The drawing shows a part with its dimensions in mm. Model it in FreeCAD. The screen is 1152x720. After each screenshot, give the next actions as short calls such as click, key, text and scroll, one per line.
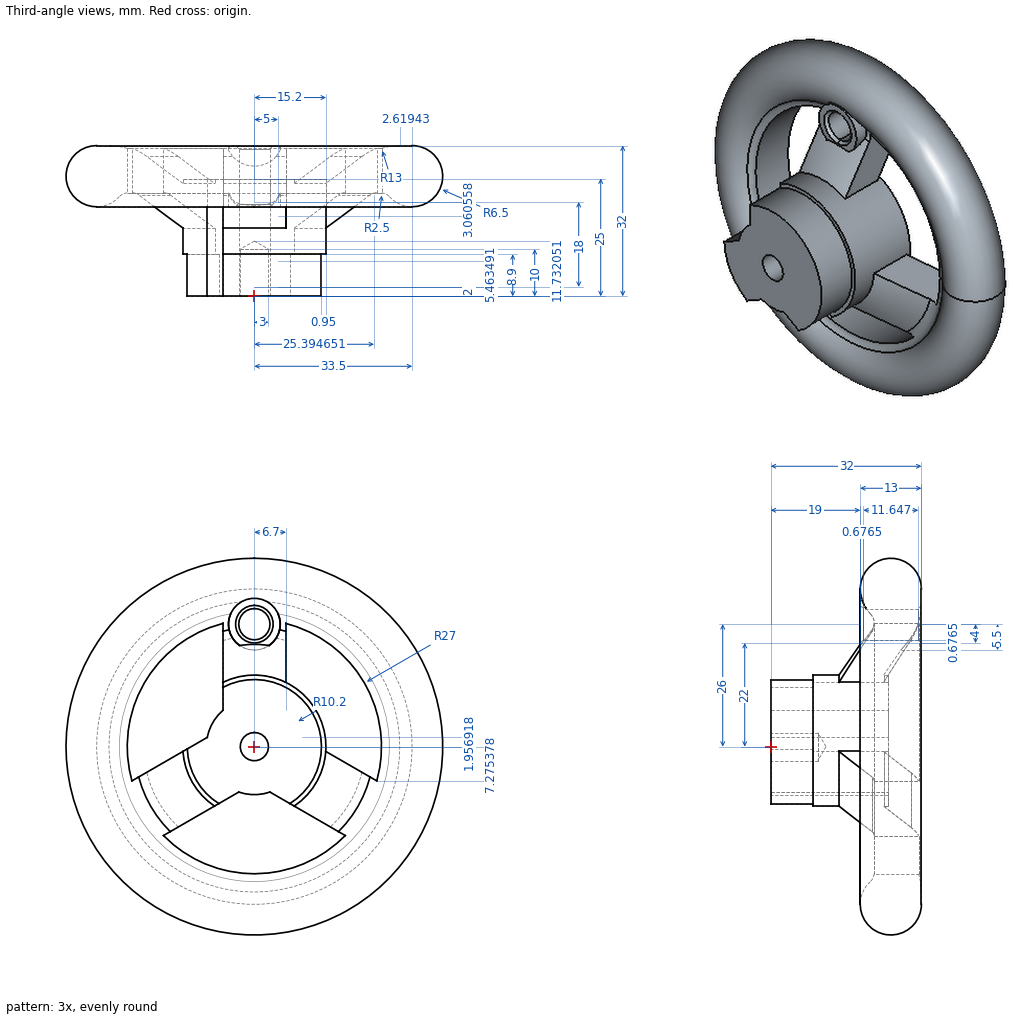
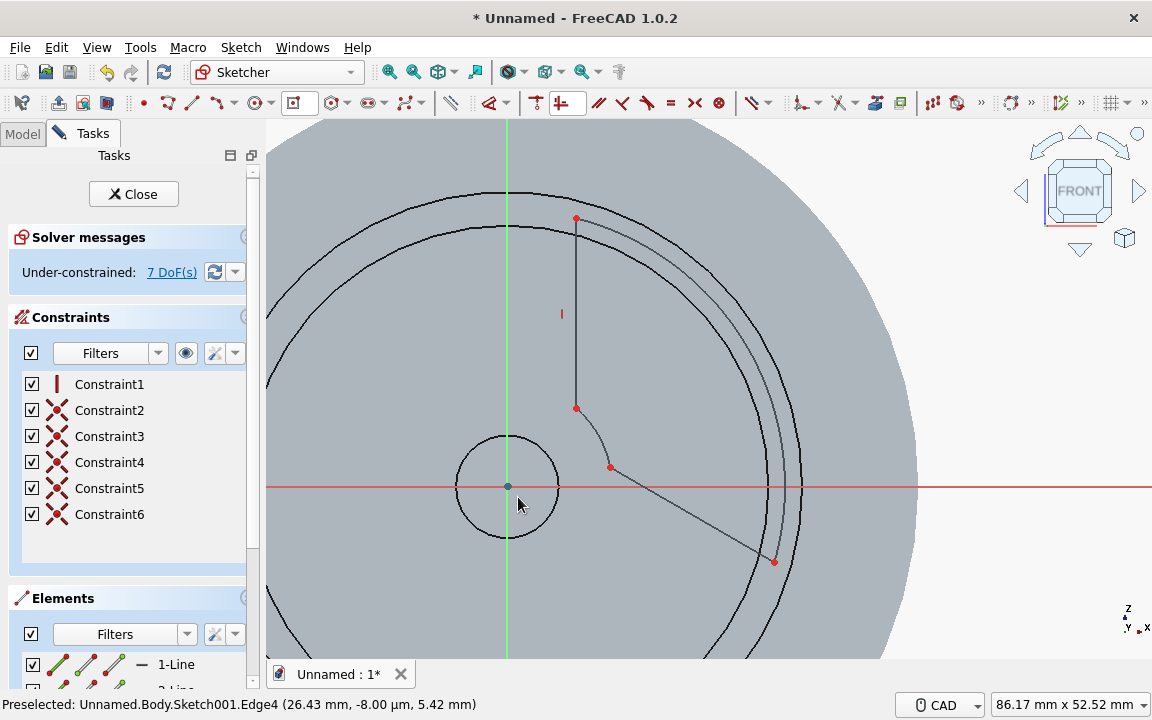
click(536, 104)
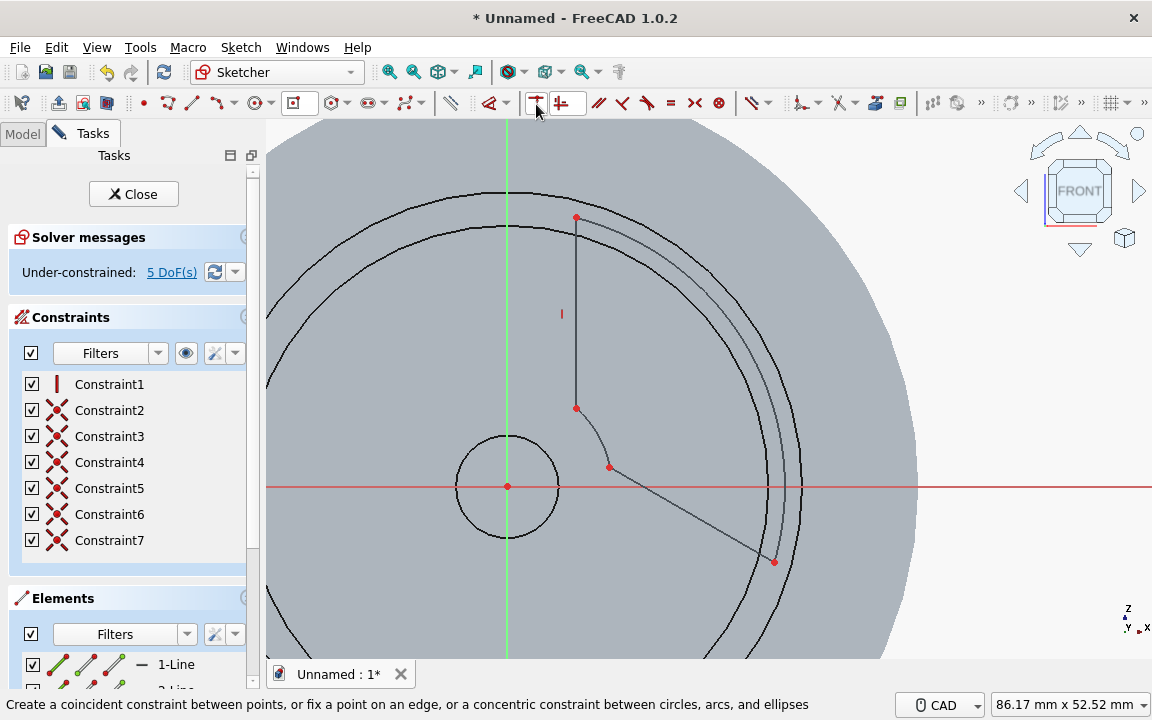
click(490, 104)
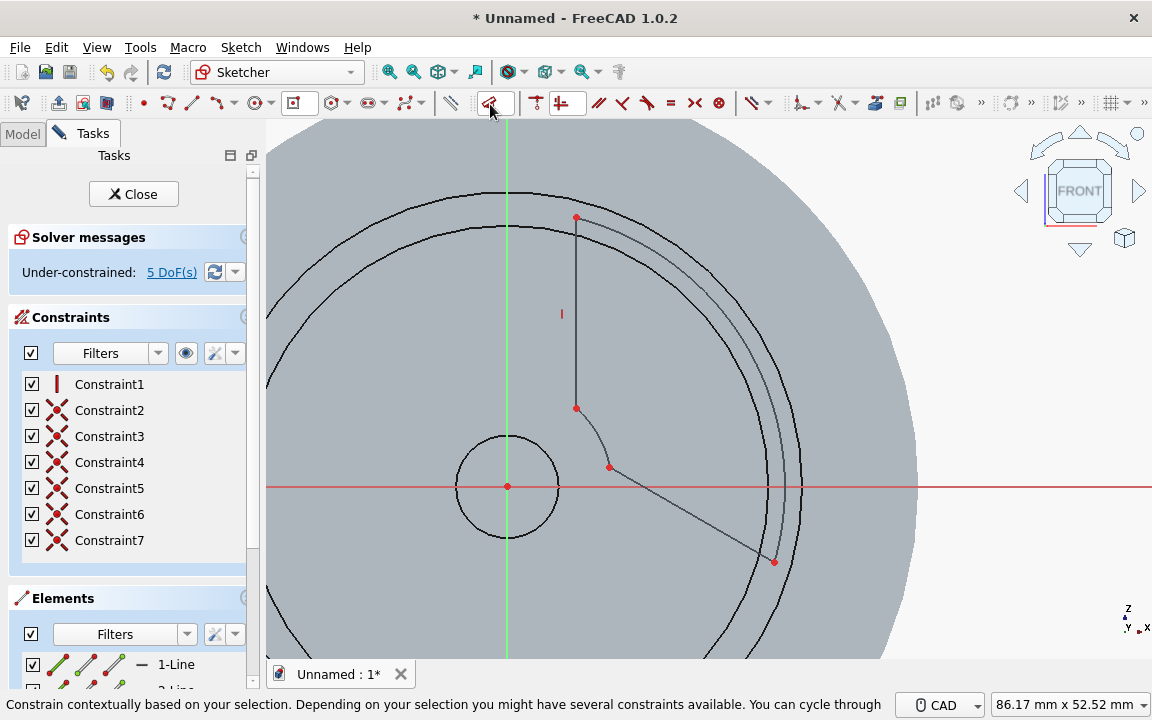
click(604, 448)
click(634, 436)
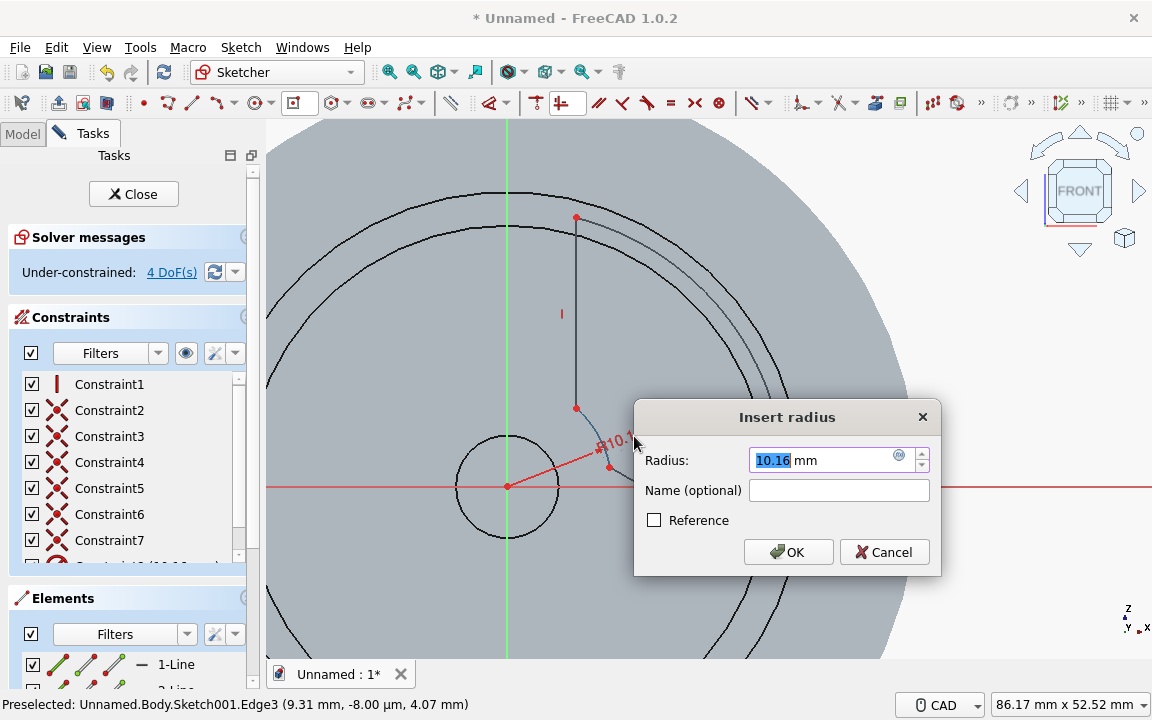
text(10.2)
key(Return)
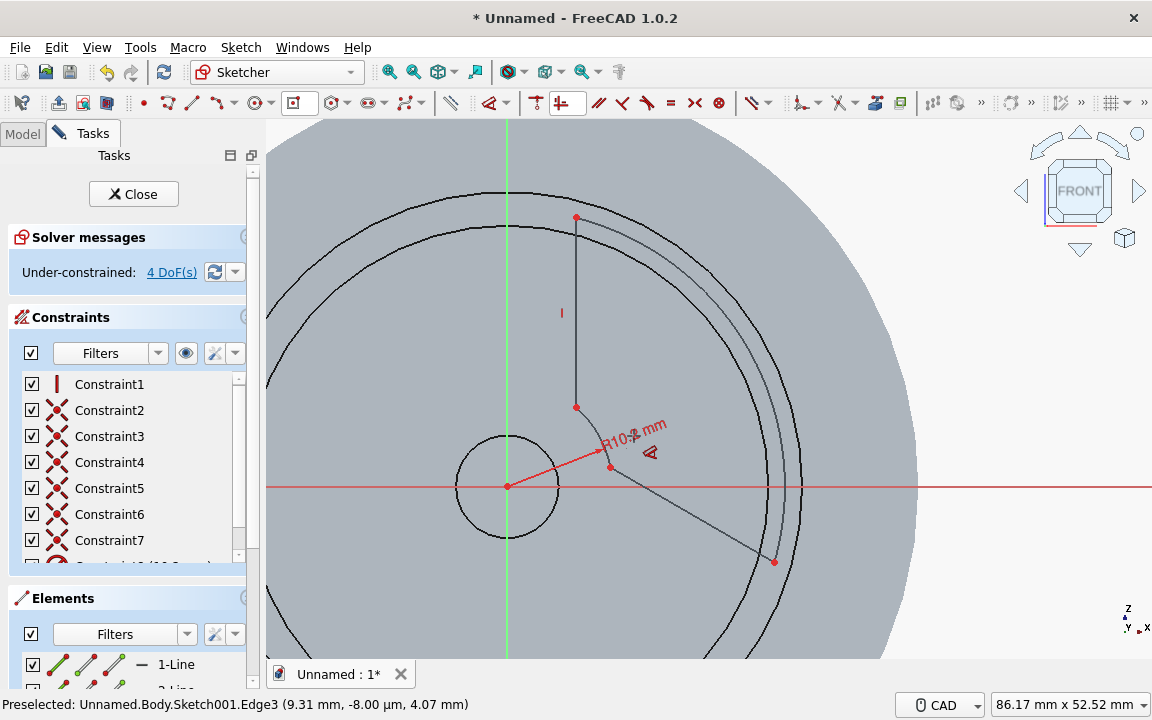
click(779, 431)
click(810, 425)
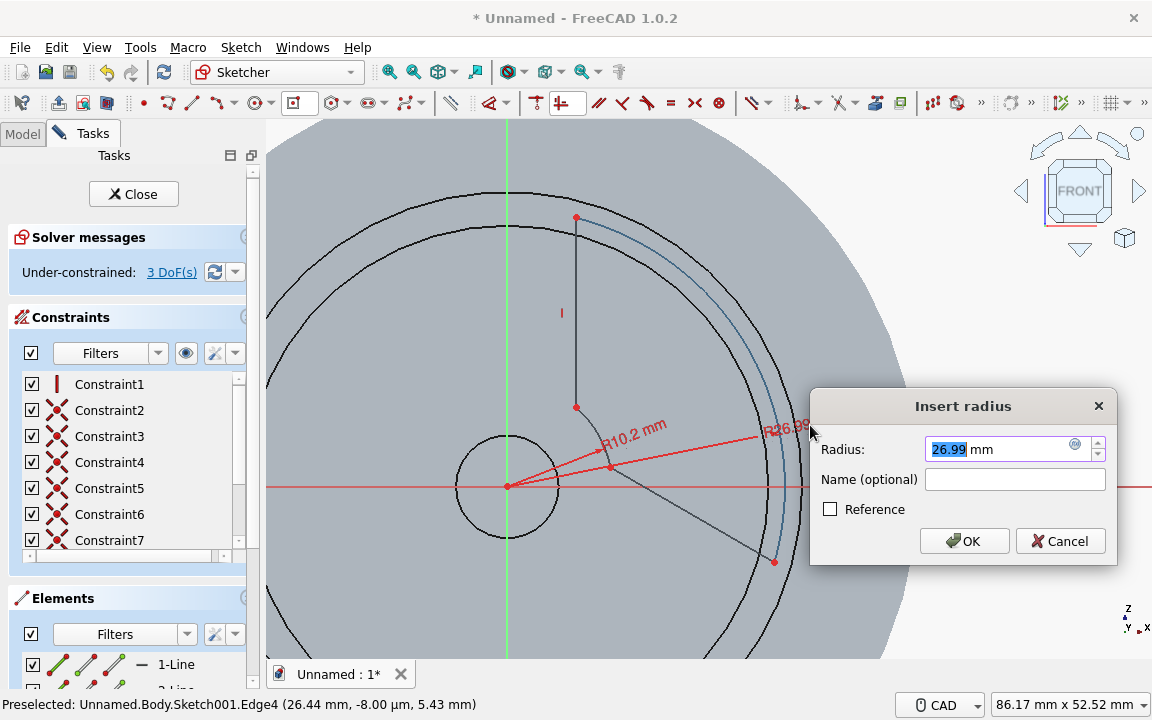
text(27)
key(Return)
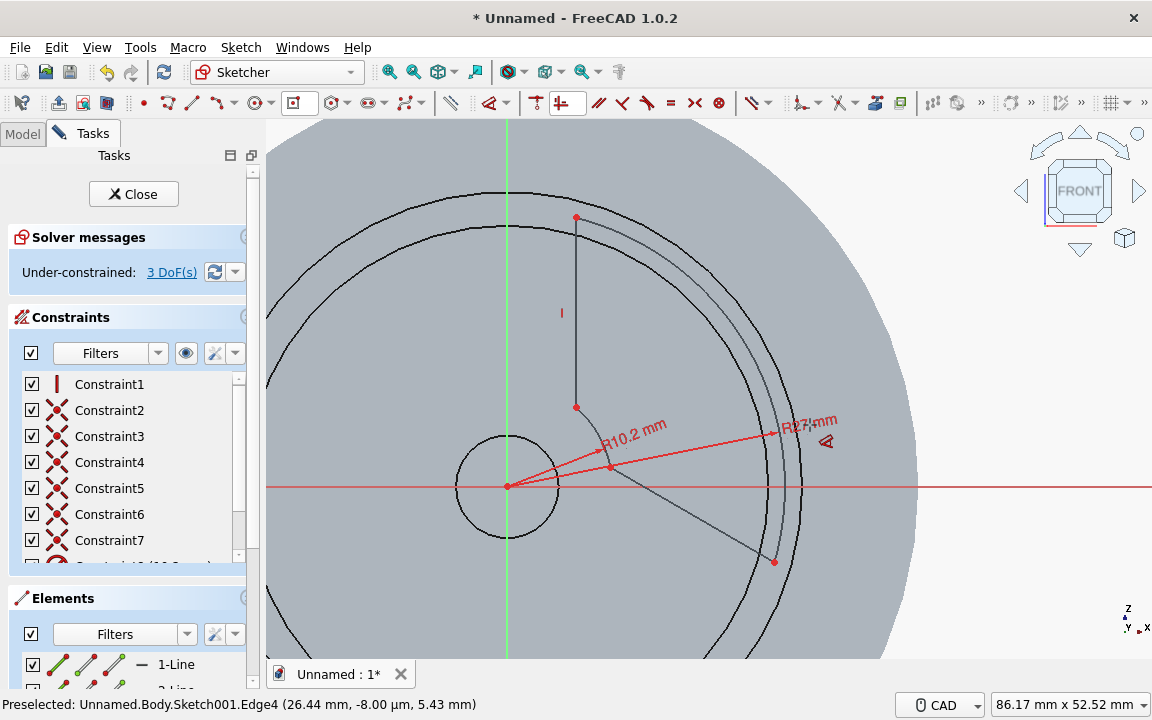
click(576, 408)
click(542, 521)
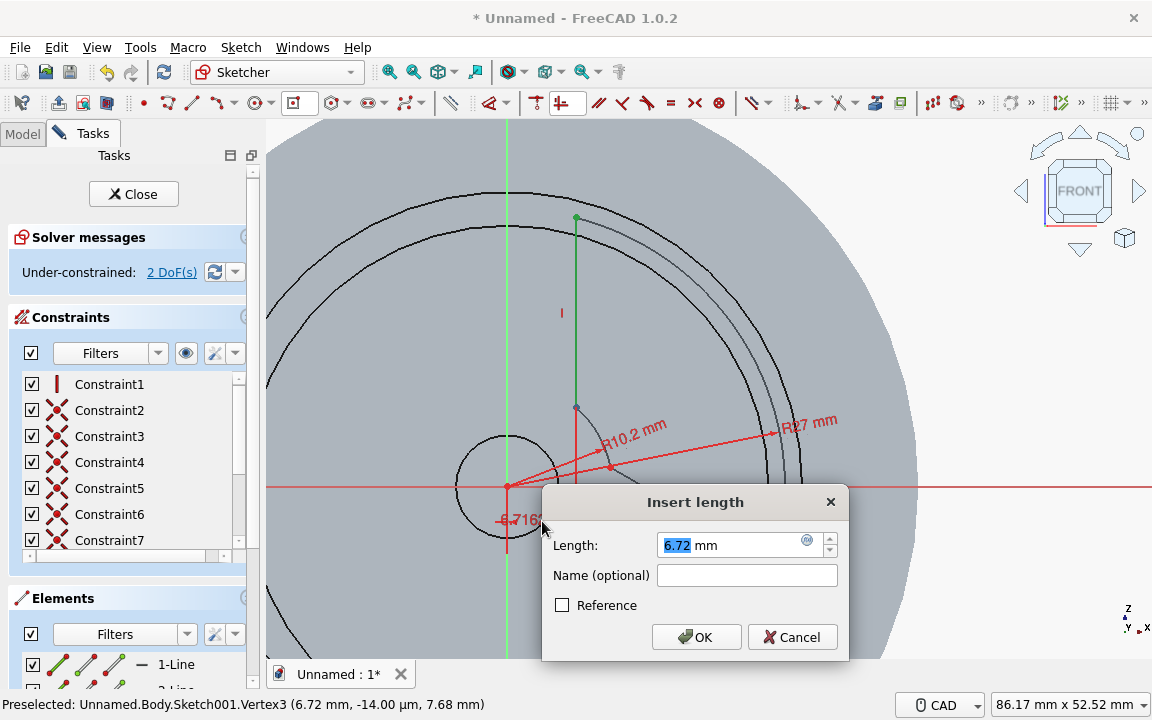
text(6.7)
key(Return)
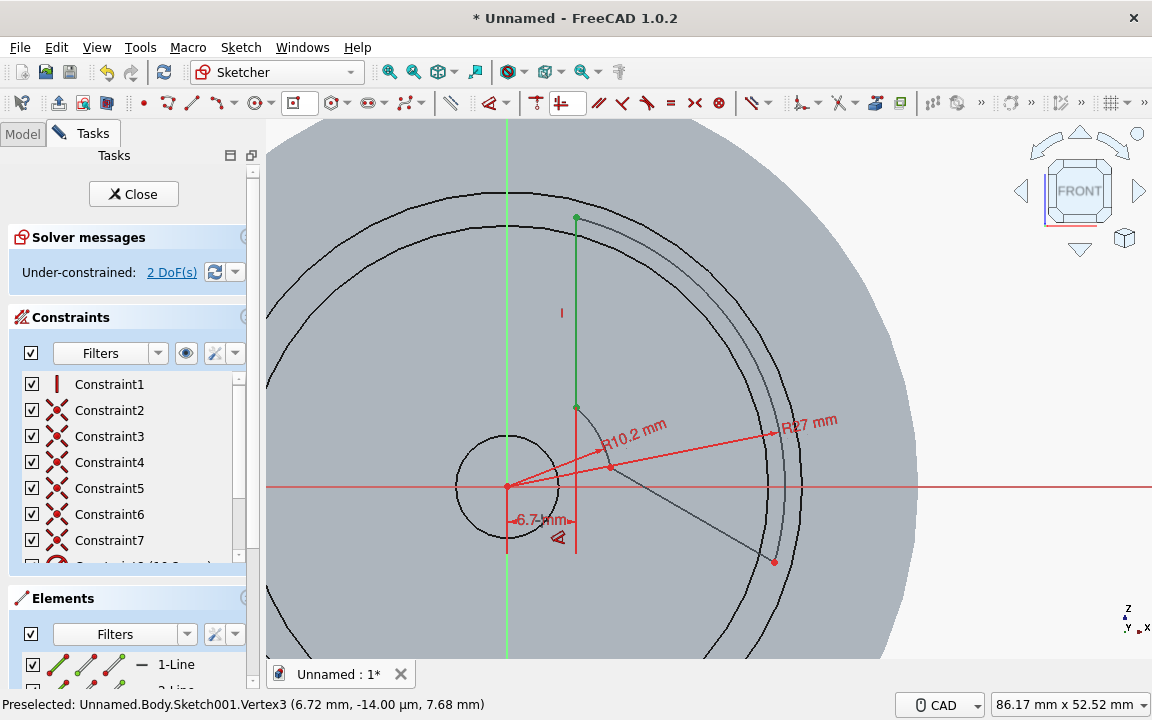
click(774, 562)
click(473, 542)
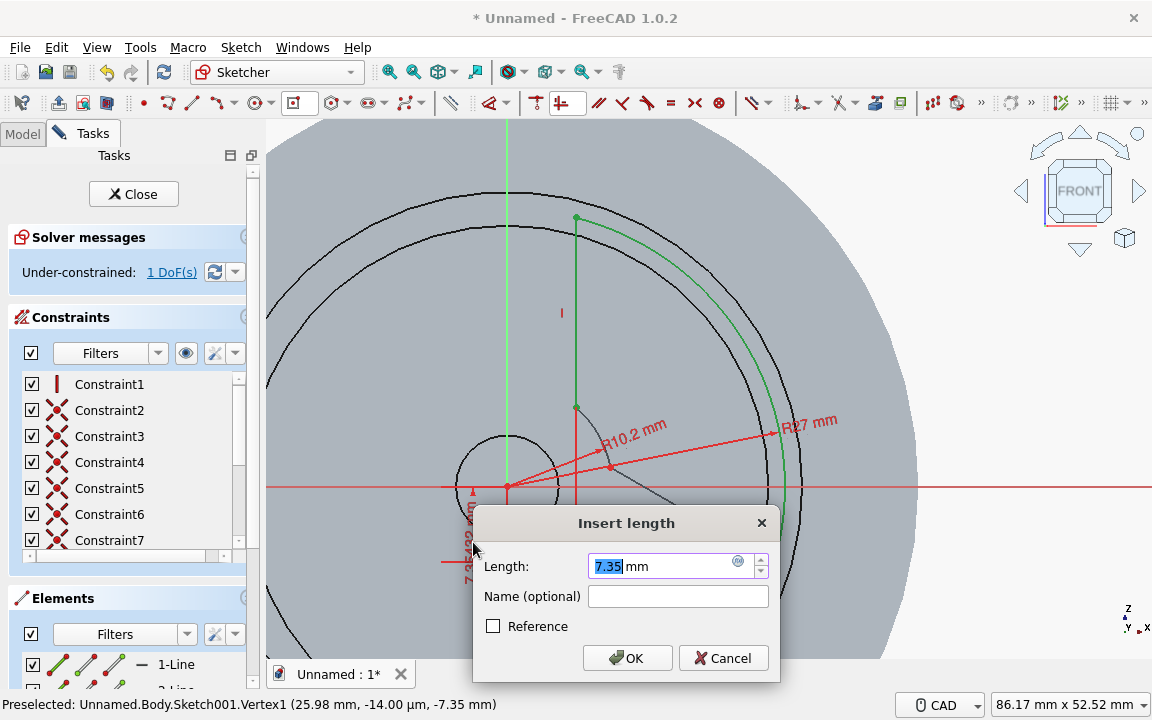
text(7.275378)
key(Return)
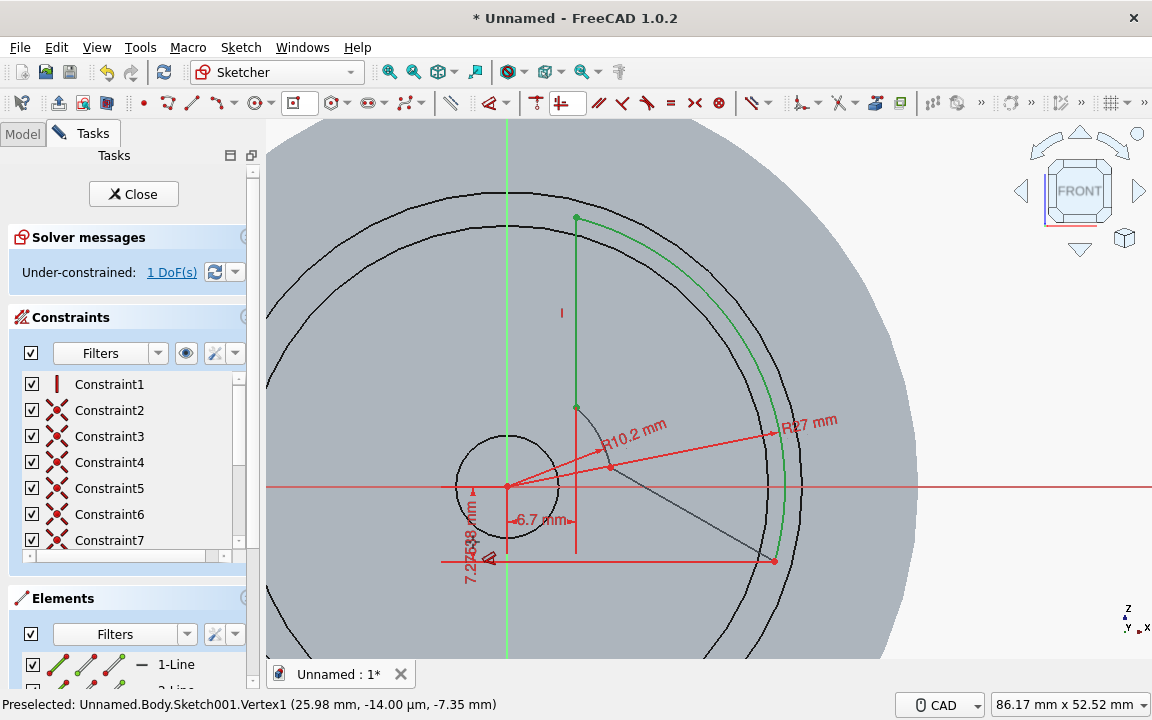
scroll(610, 467, up, 4)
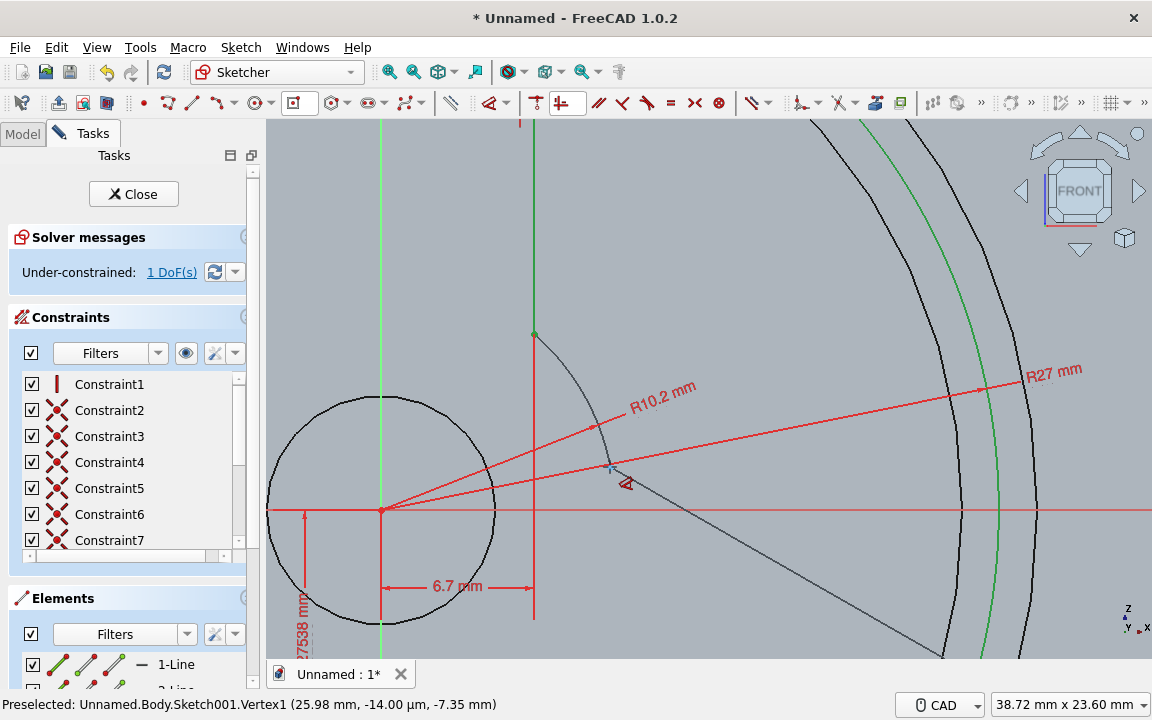
click(610, 467)
click(347, 489)